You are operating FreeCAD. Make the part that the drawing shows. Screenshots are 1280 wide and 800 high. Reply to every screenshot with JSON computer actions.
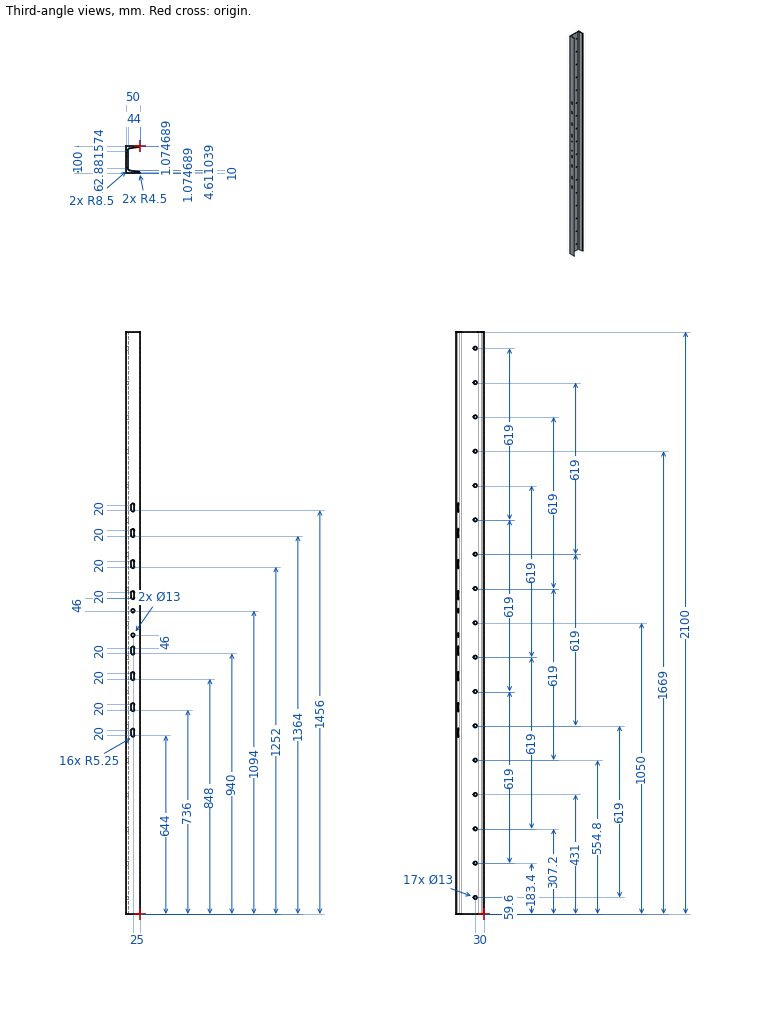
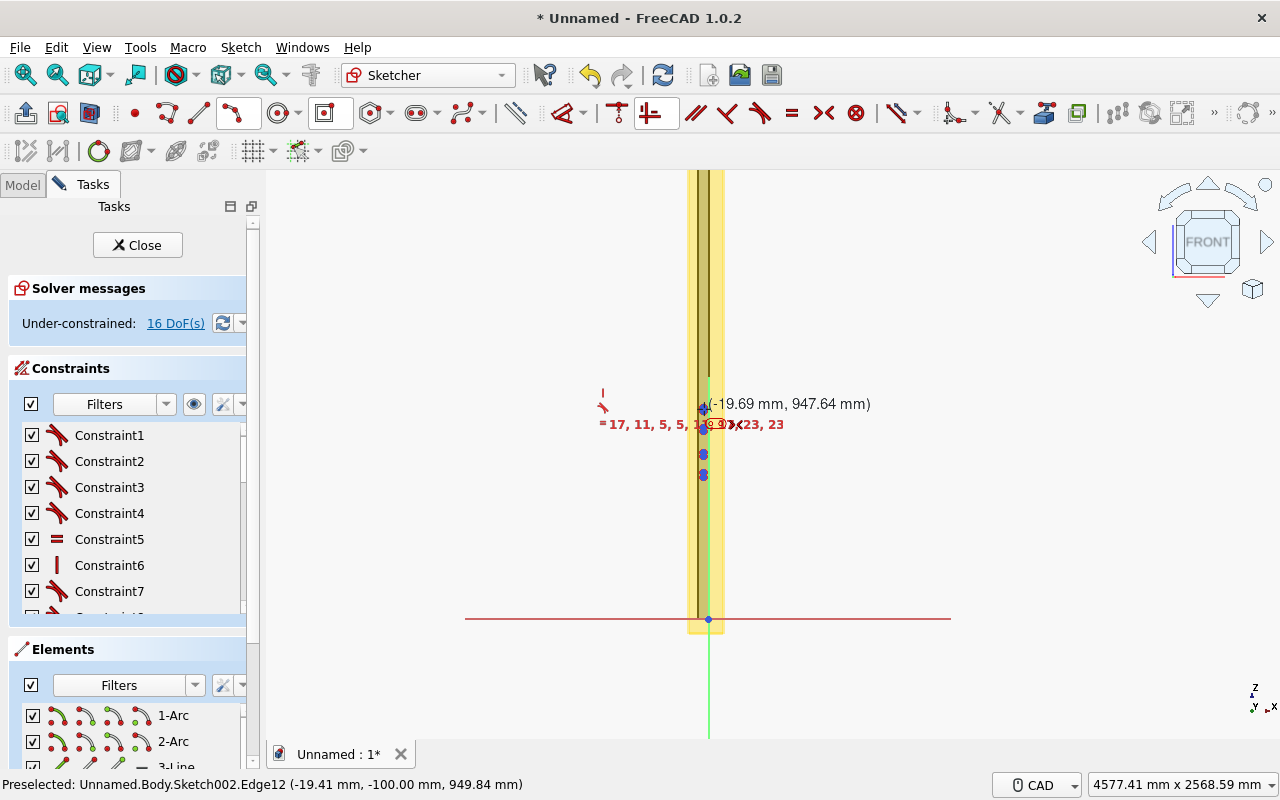
{"action": "scroll", "coordinate": [703, 342], "scroll_direction": "up", "scroll_amount": 15}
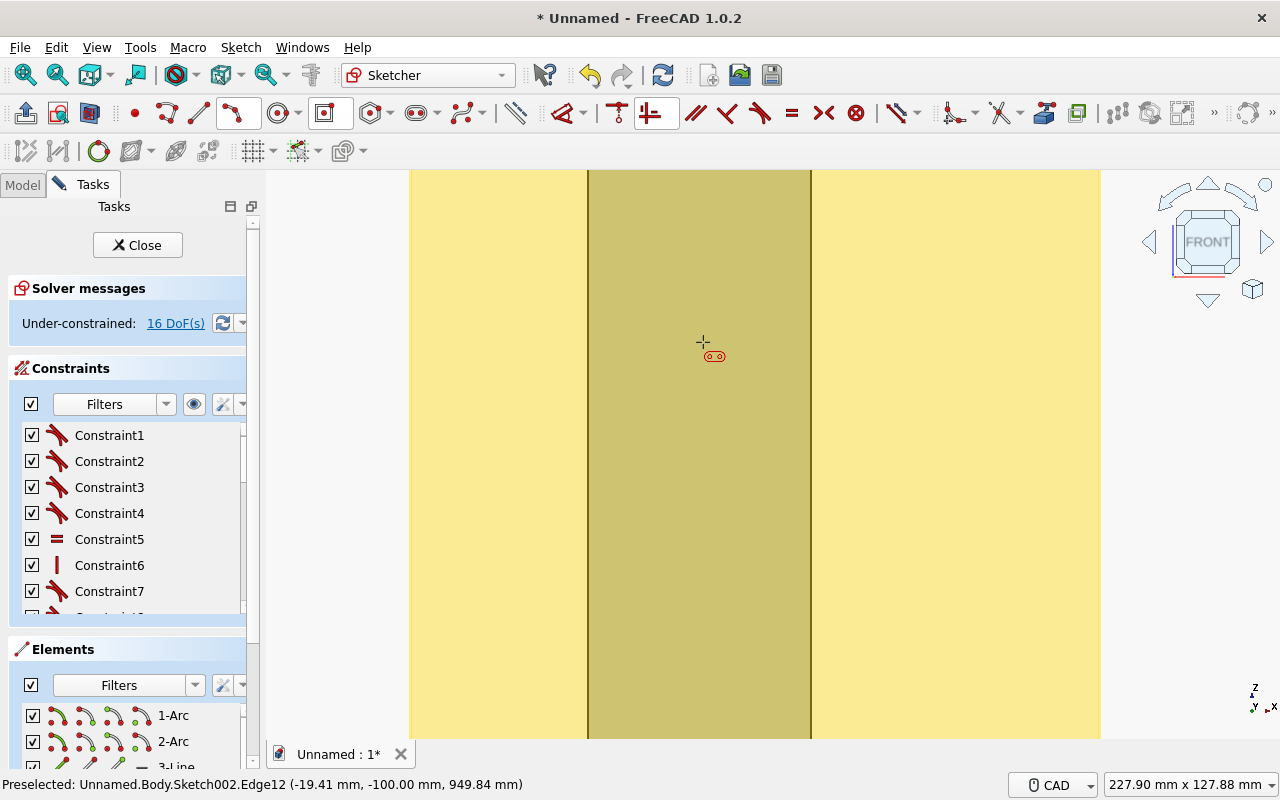
{"action": "scroll", "coordinate": [703, 341], "scroll_direction": "down", "scroll_amount": 15}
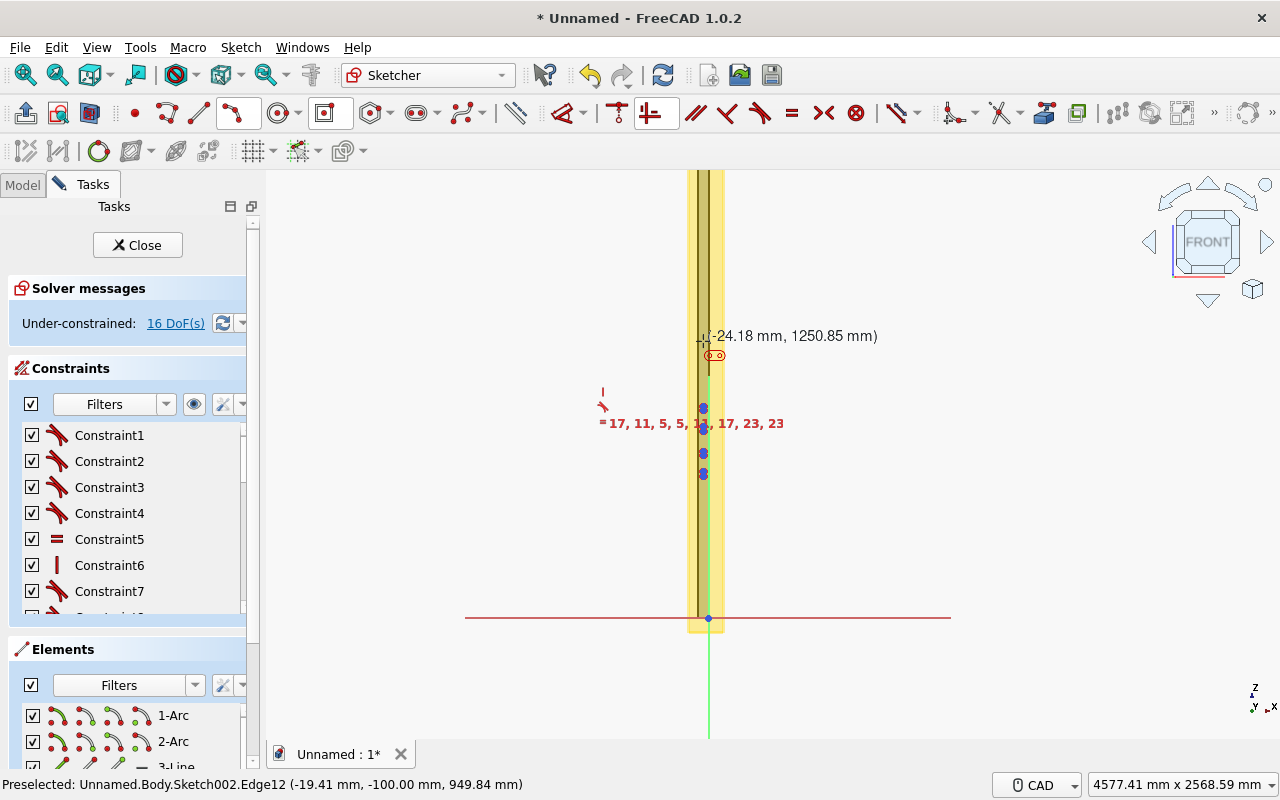
{"action": "scroll", "coordinate": [703, 341], "scroll_direction": "up", "scroll_amount": 6}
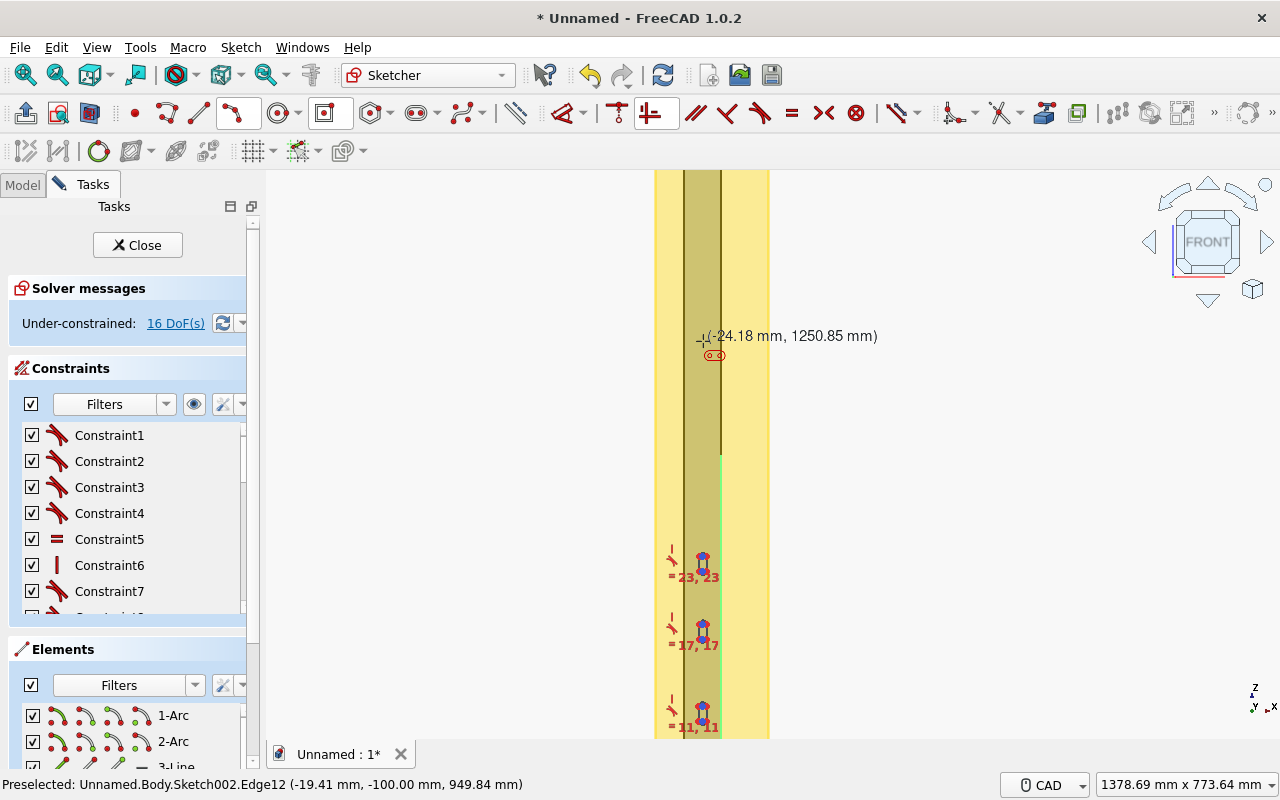
{"action": "left_click", "coordinate": [703, 341]}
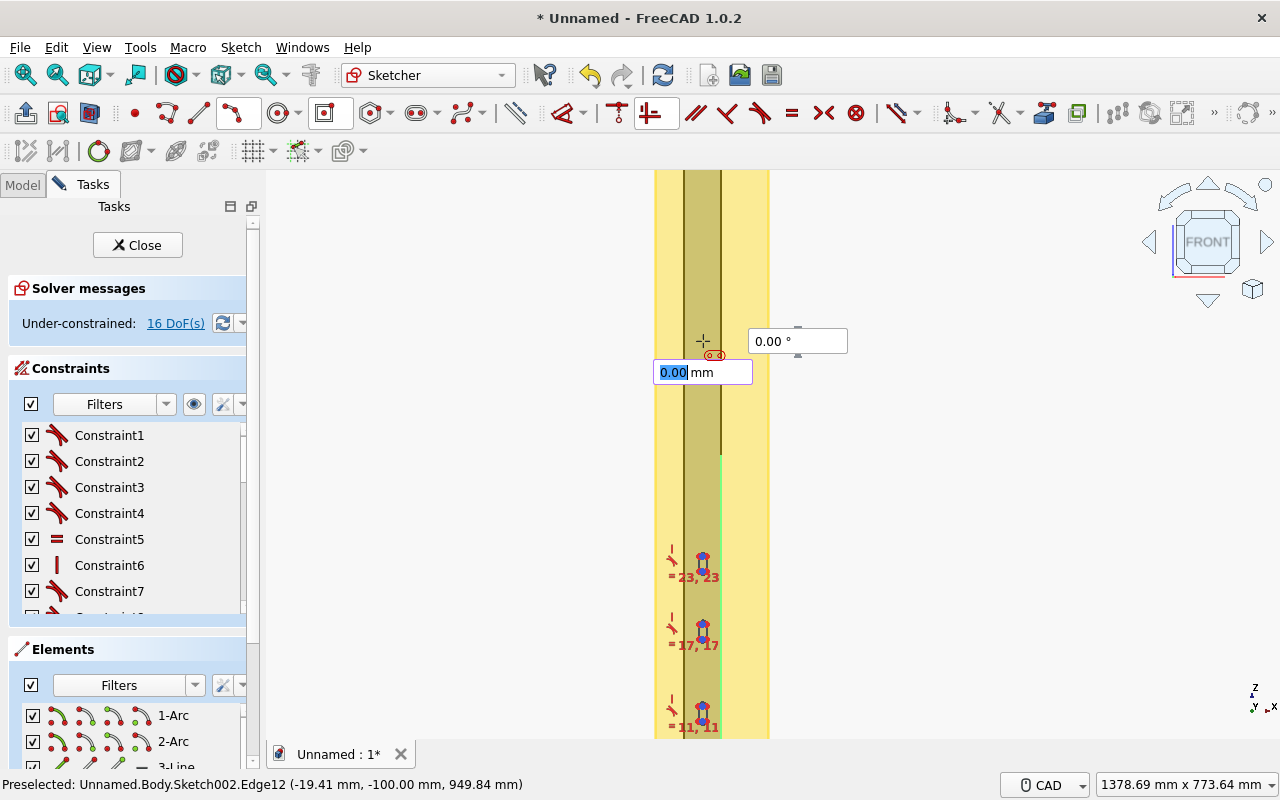
{"action": "left_click", "coordinate": [703, 326]}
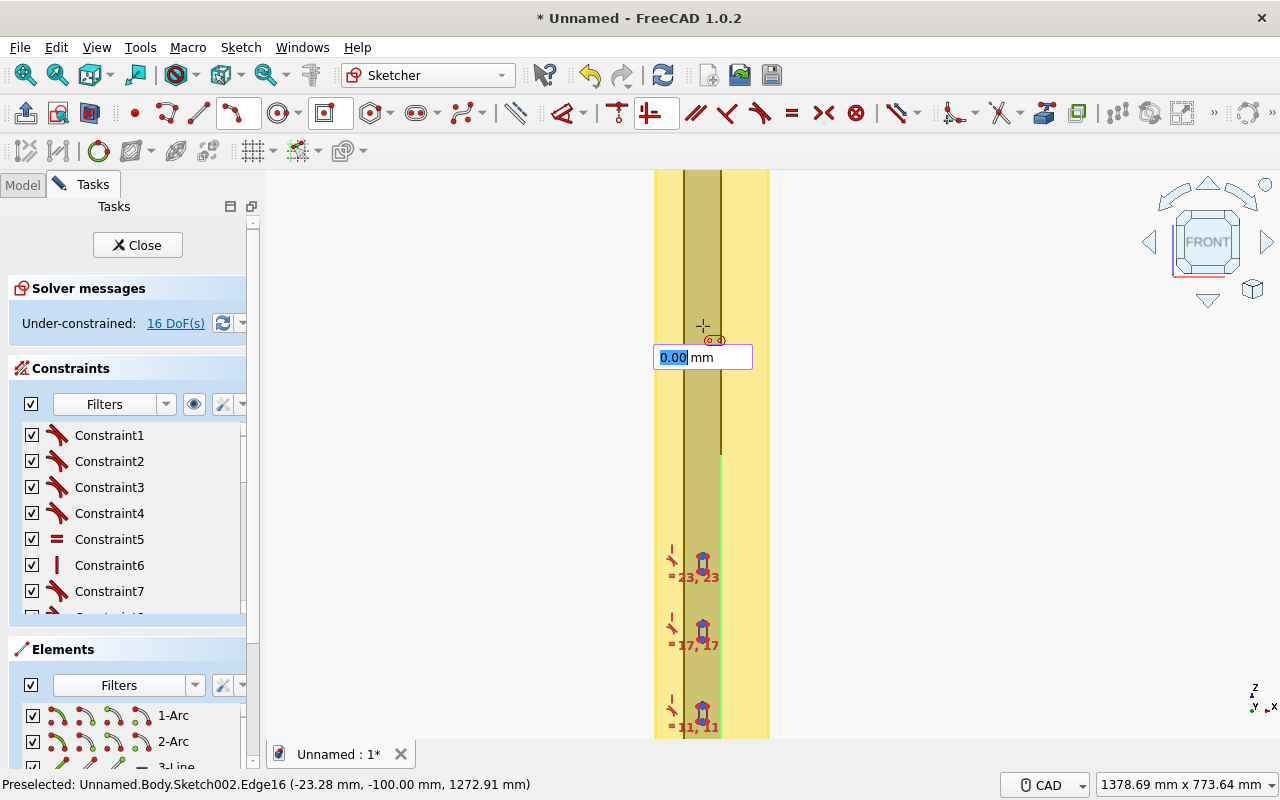
{"action": "scroll", "coordinate": [707, 333], "scroll_direction": "up", "scroll_amount": 8}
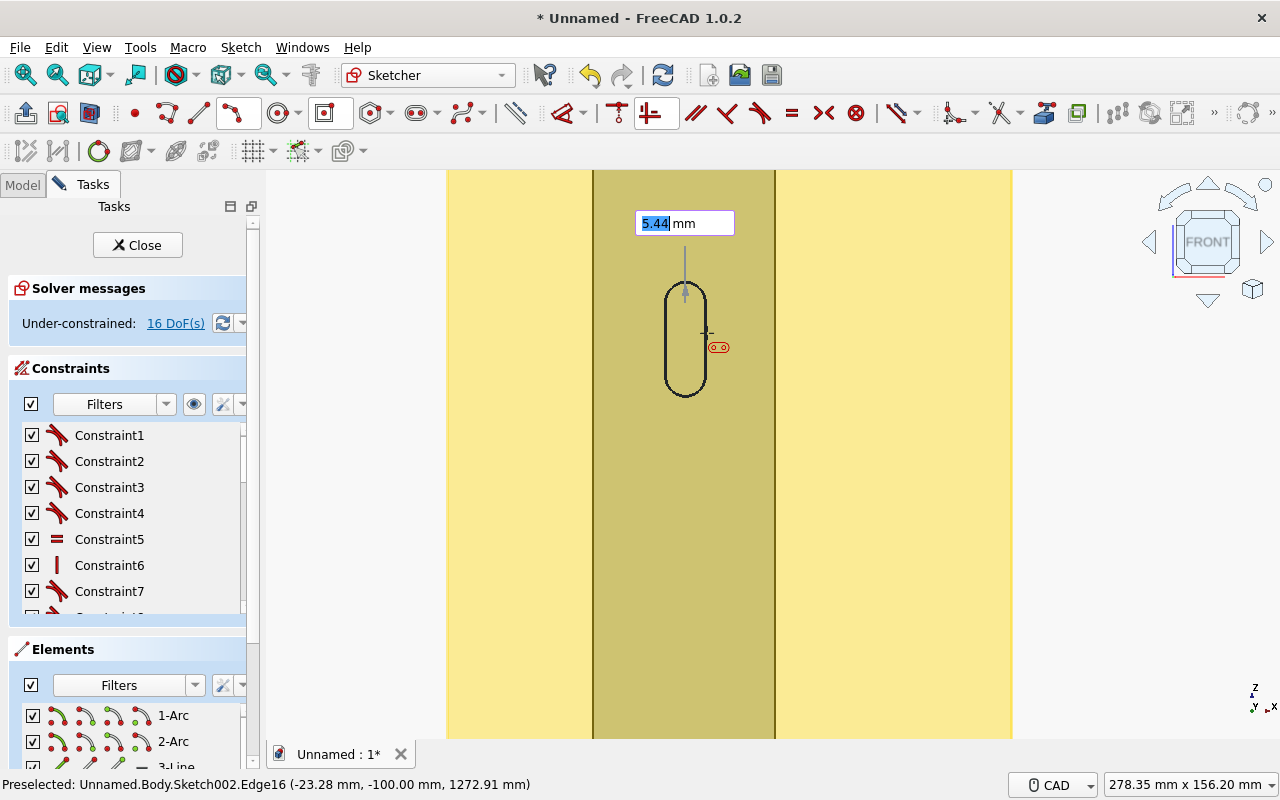
{"action": "left_click", "coordinate": [703, 333]}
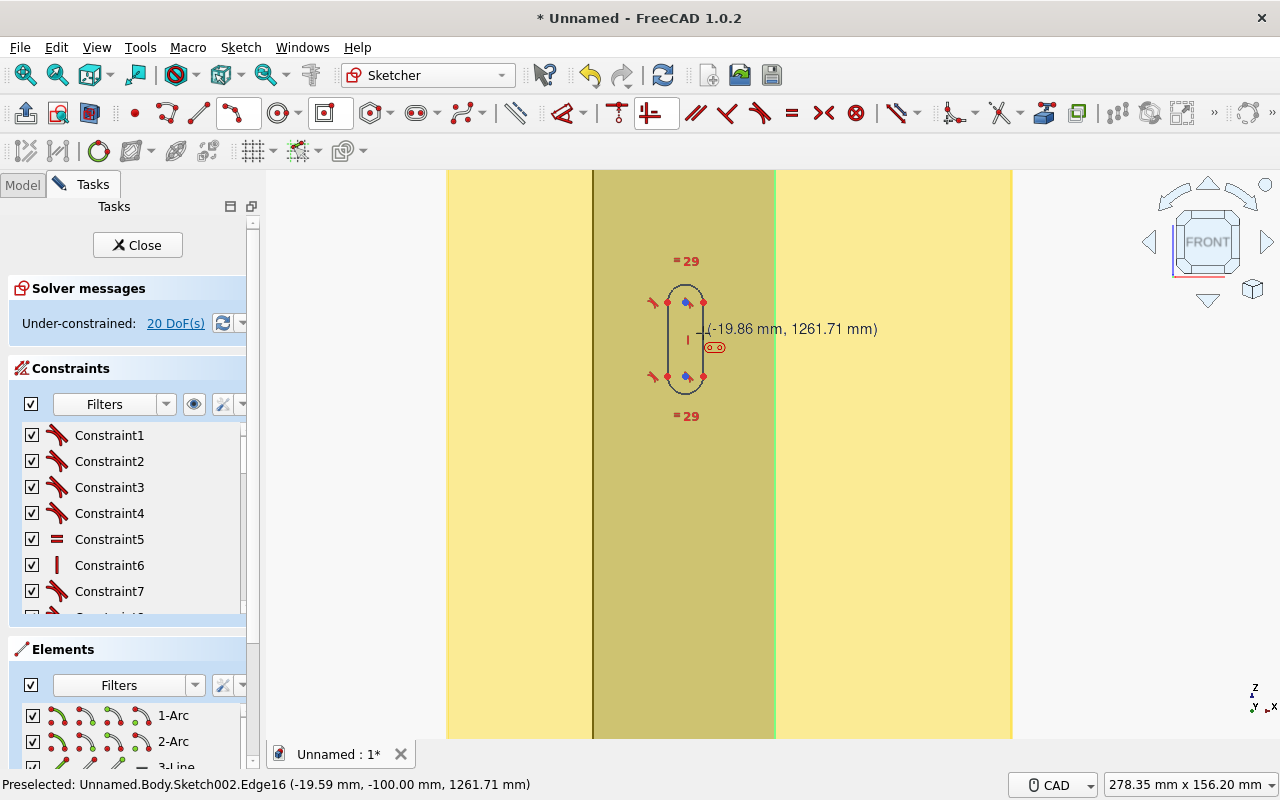
{"action": "scroll", "coordinate": [704, 339], "scroll_direction": "down", "scroll_amount": 14}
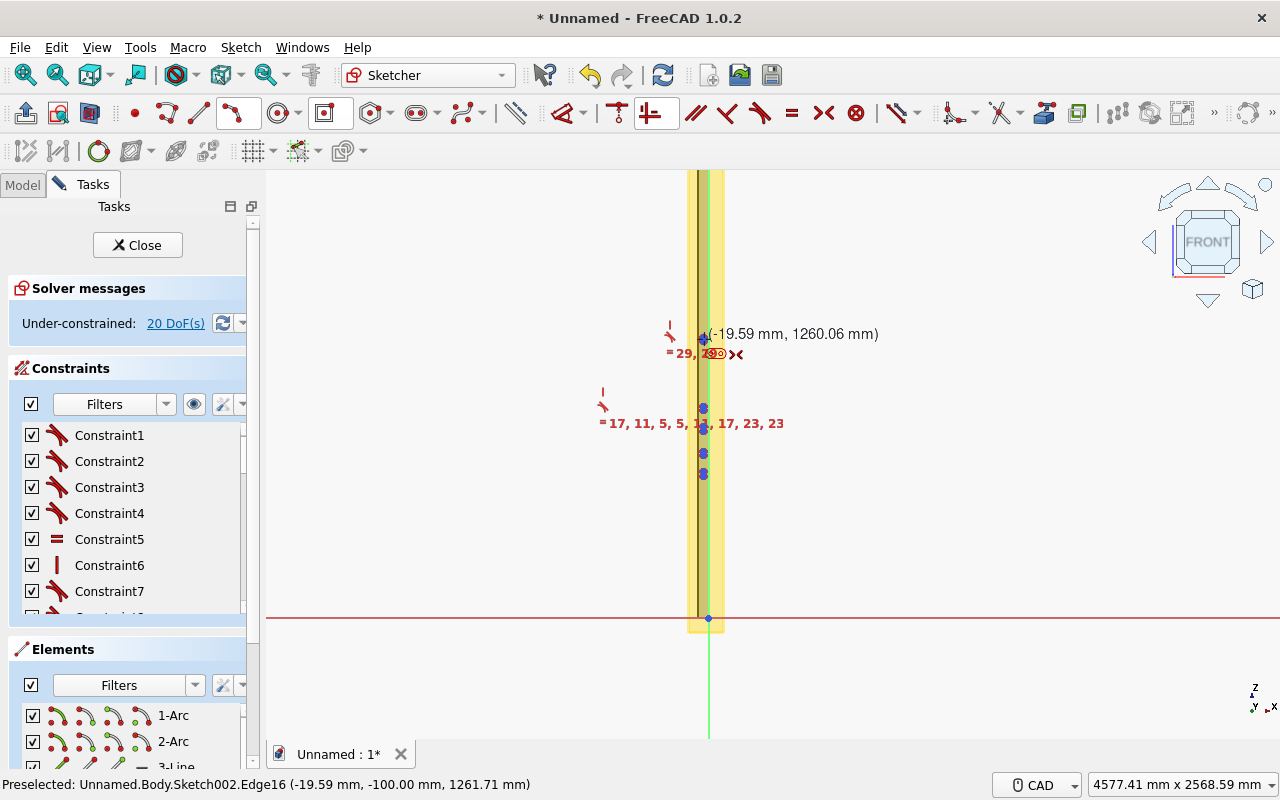
{"action": "scroll", "coordinate": [703, 296], "scroll_direction": "up", "scroll_amount": 15}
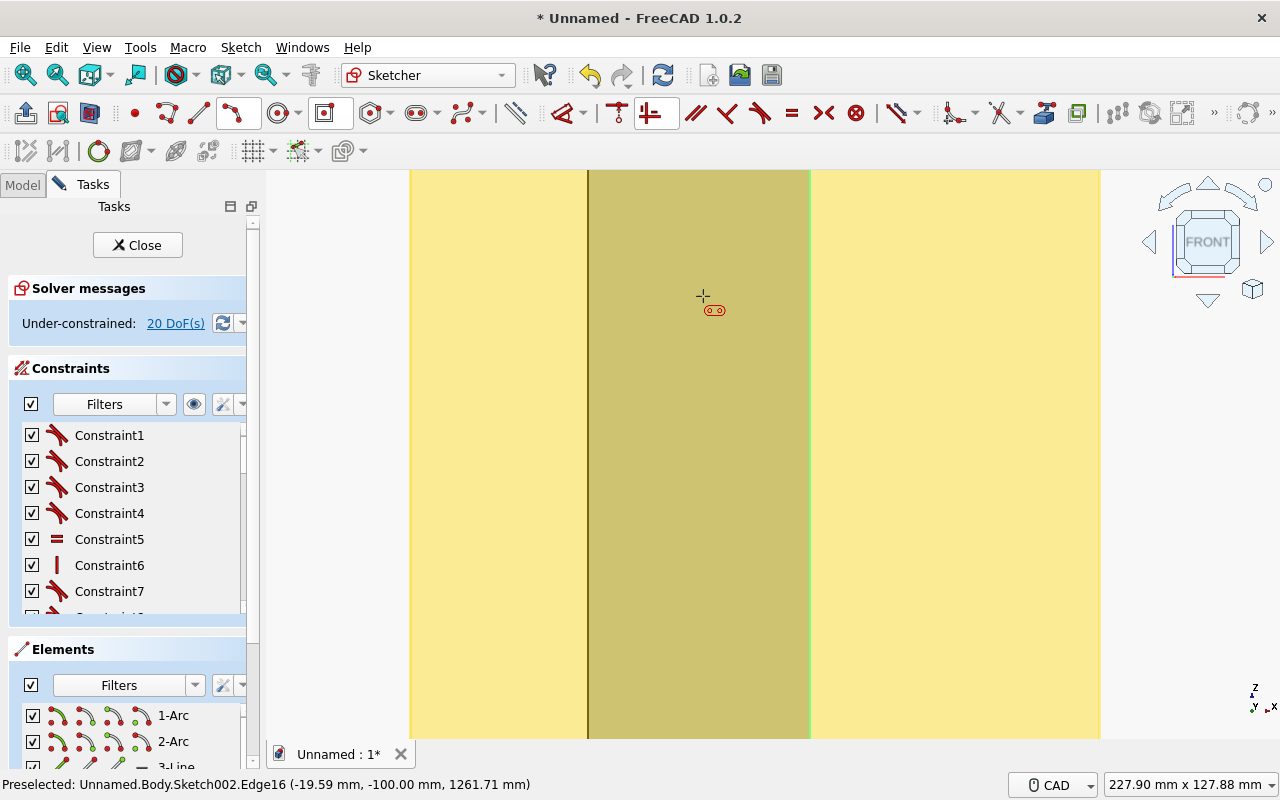
{"action": "scroll", "coordinate": [703, 296], "scroll_direction": "down", "scroll_amount": 15}